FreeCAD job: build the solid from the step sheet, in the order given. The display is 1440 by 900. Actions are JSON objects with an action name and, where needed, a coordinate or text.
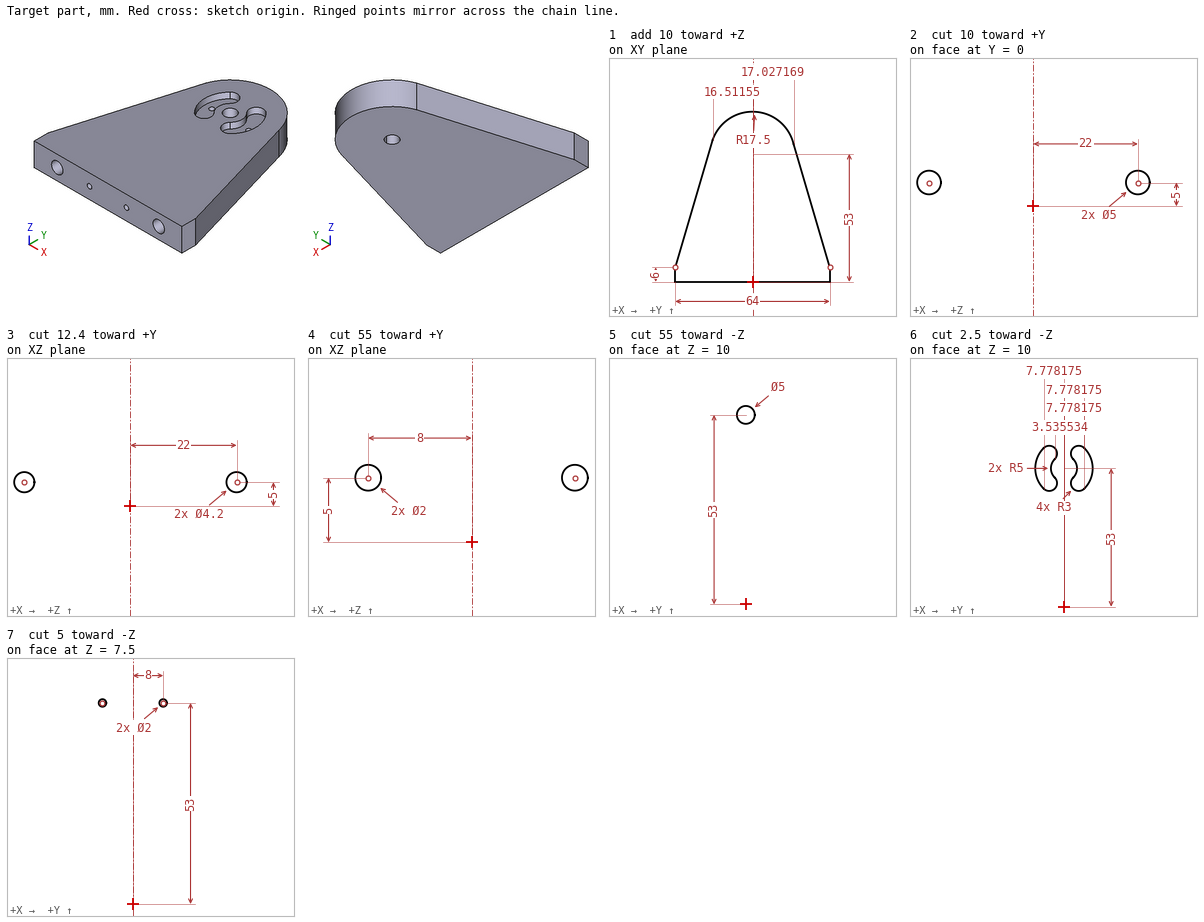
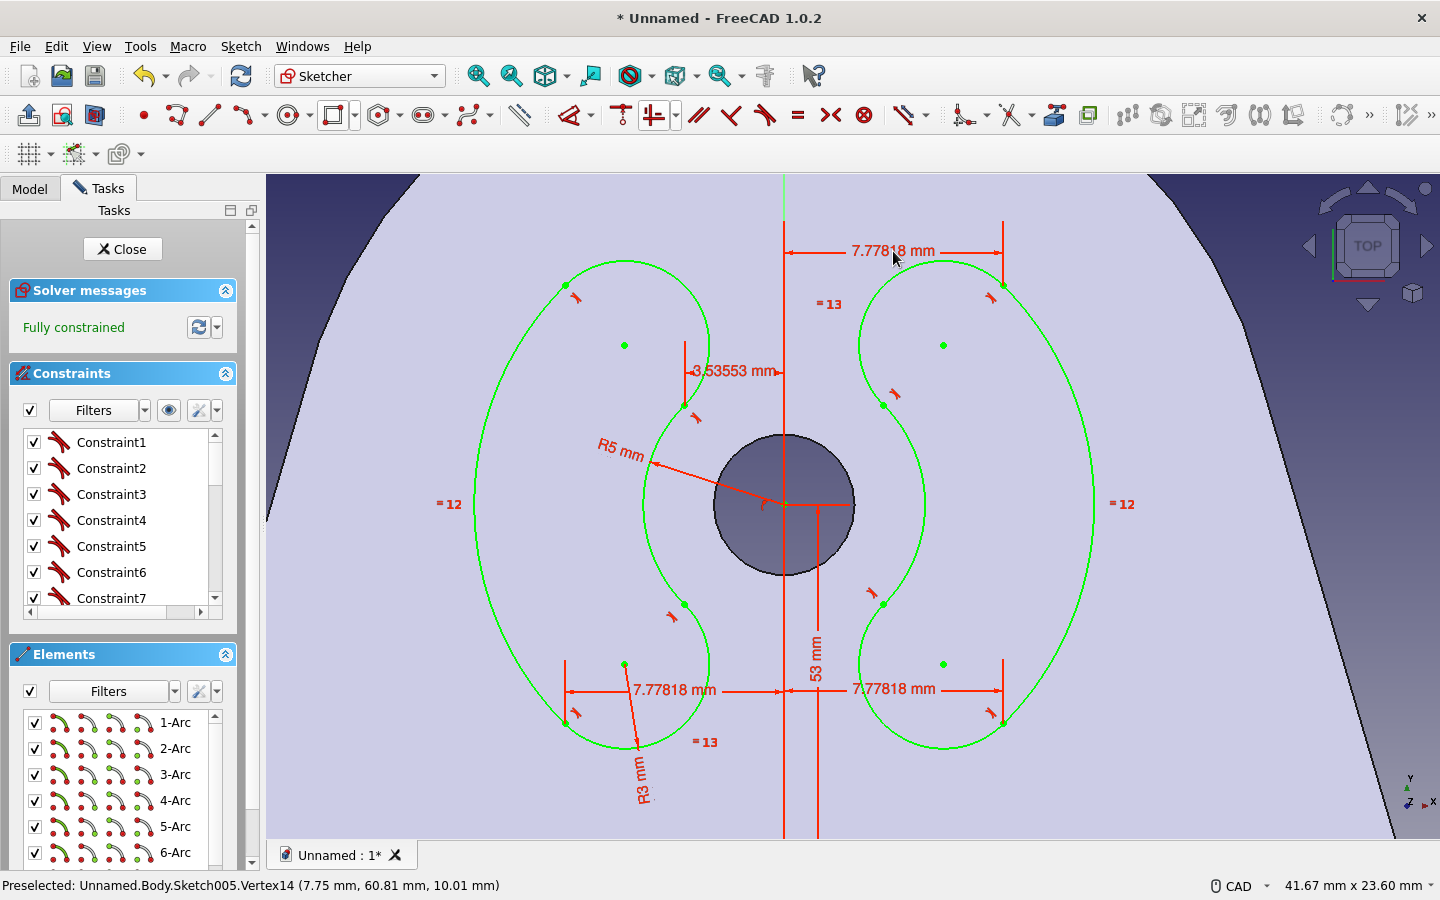
{"action": "left_click", "coordinate": [123, 249]}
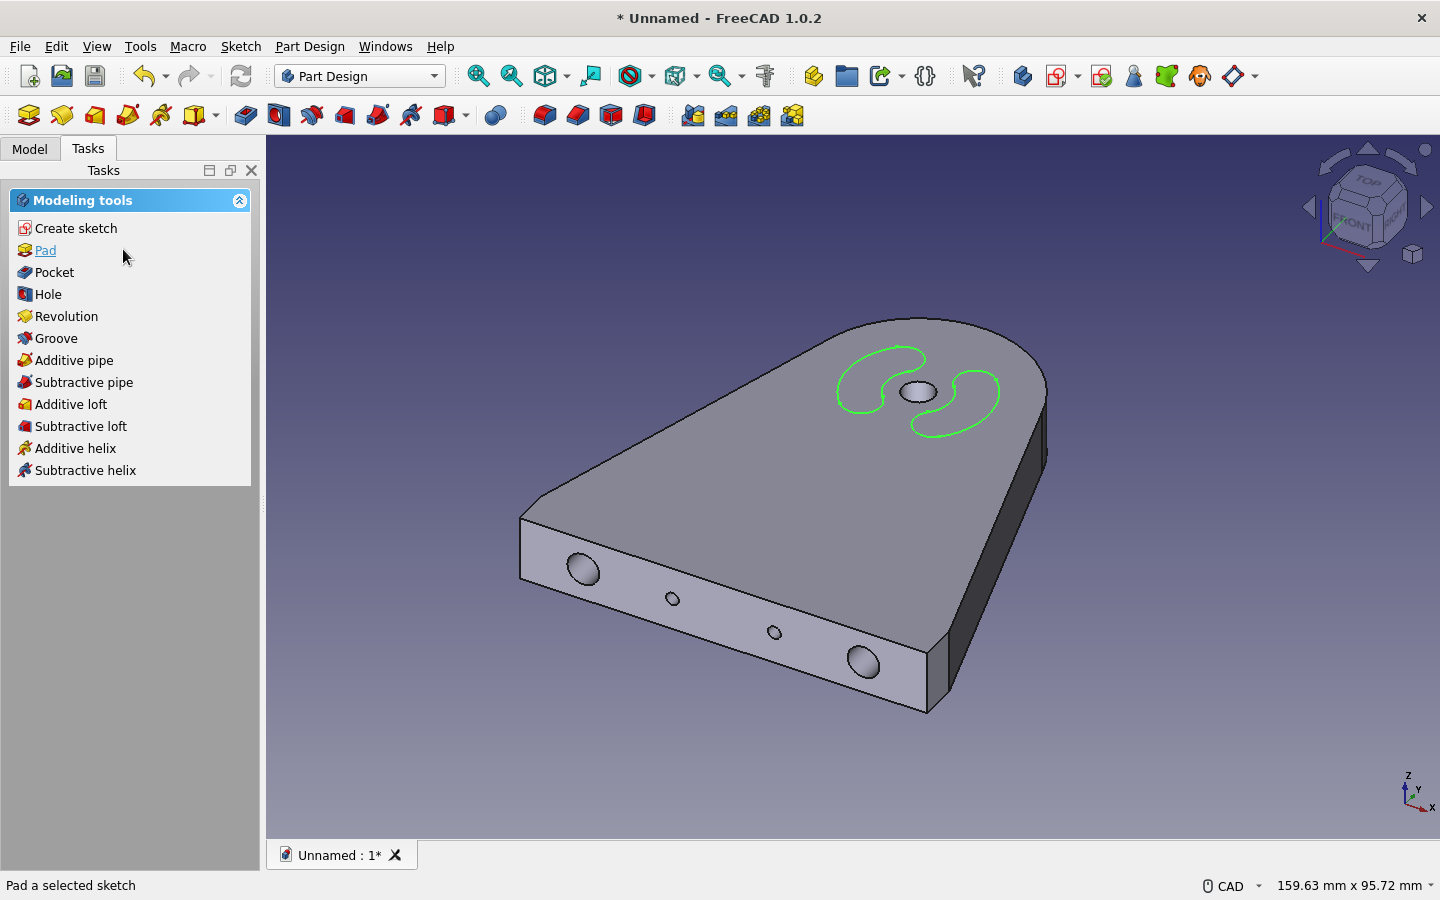
{"action": "left_click", "coordinate": [246, 116]}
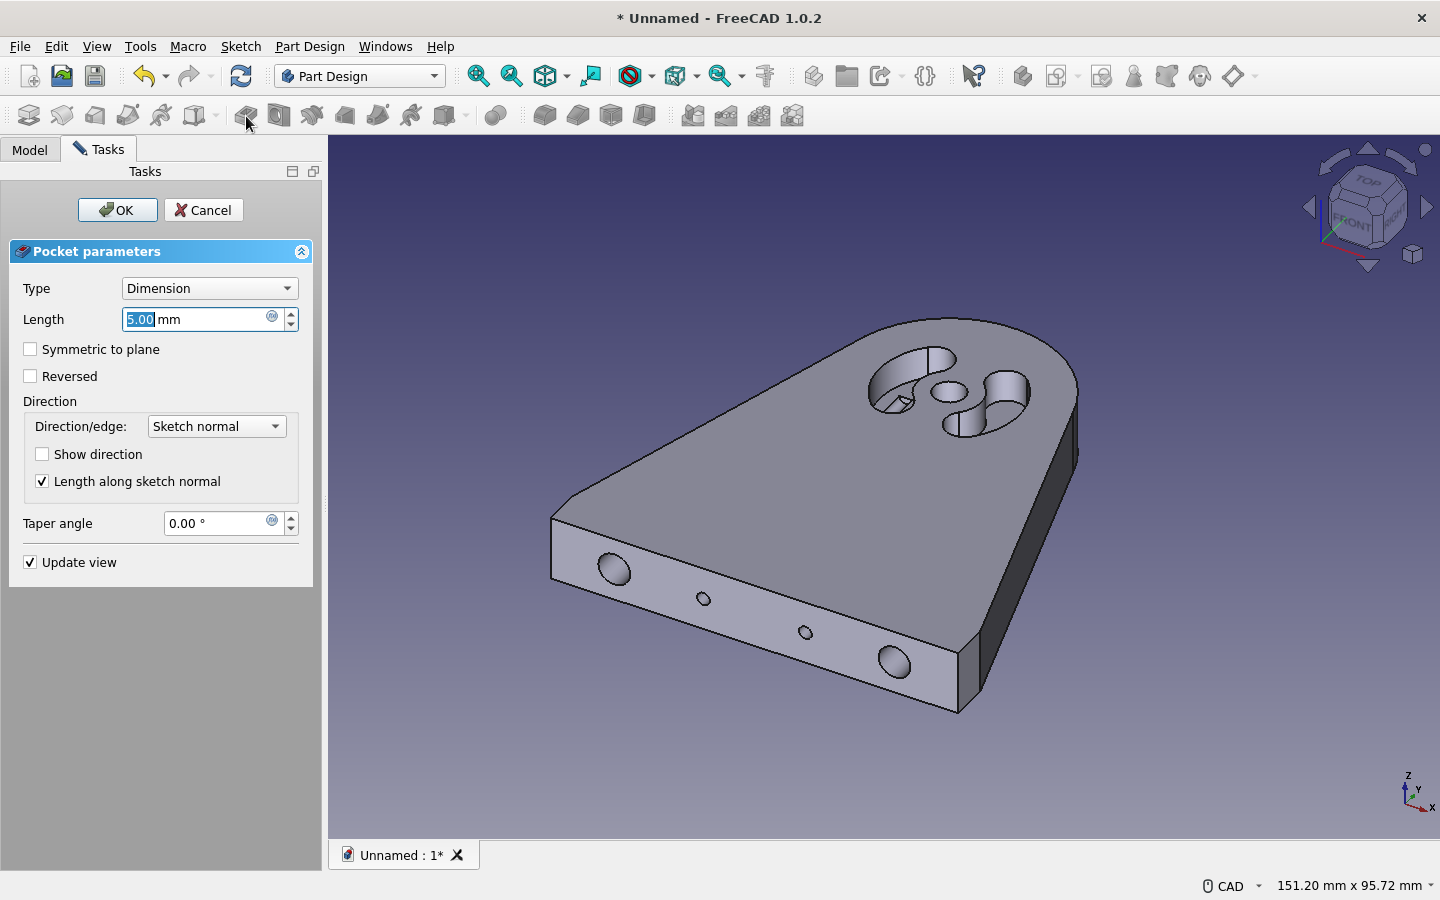
{"action": "type", "text": "2.5"}
{"action": "key", "text": "Tab"}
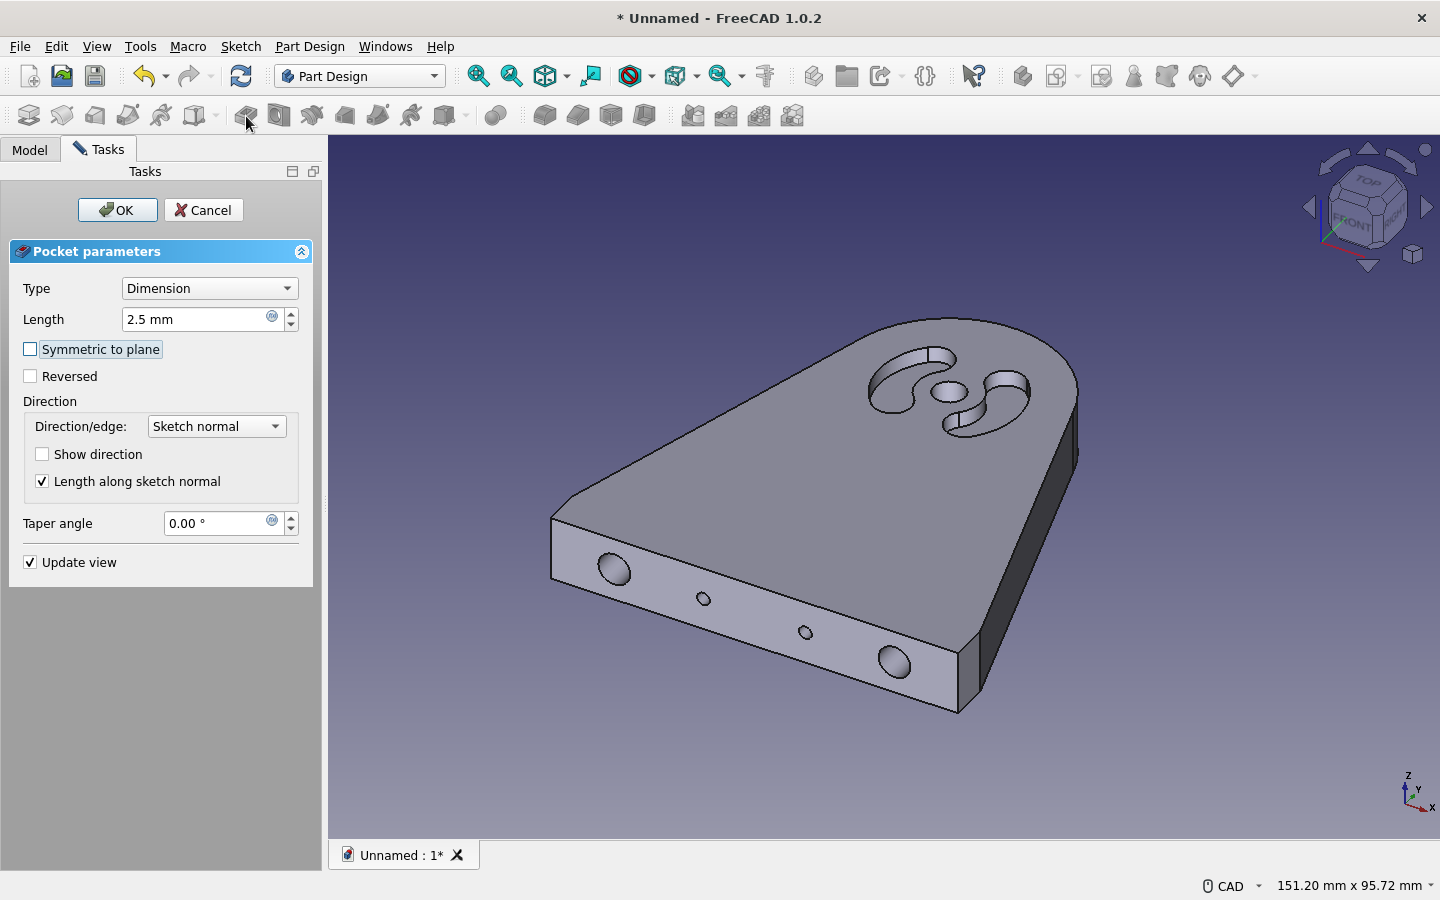
{"action": "left_click", "coordinate": [118, 210]}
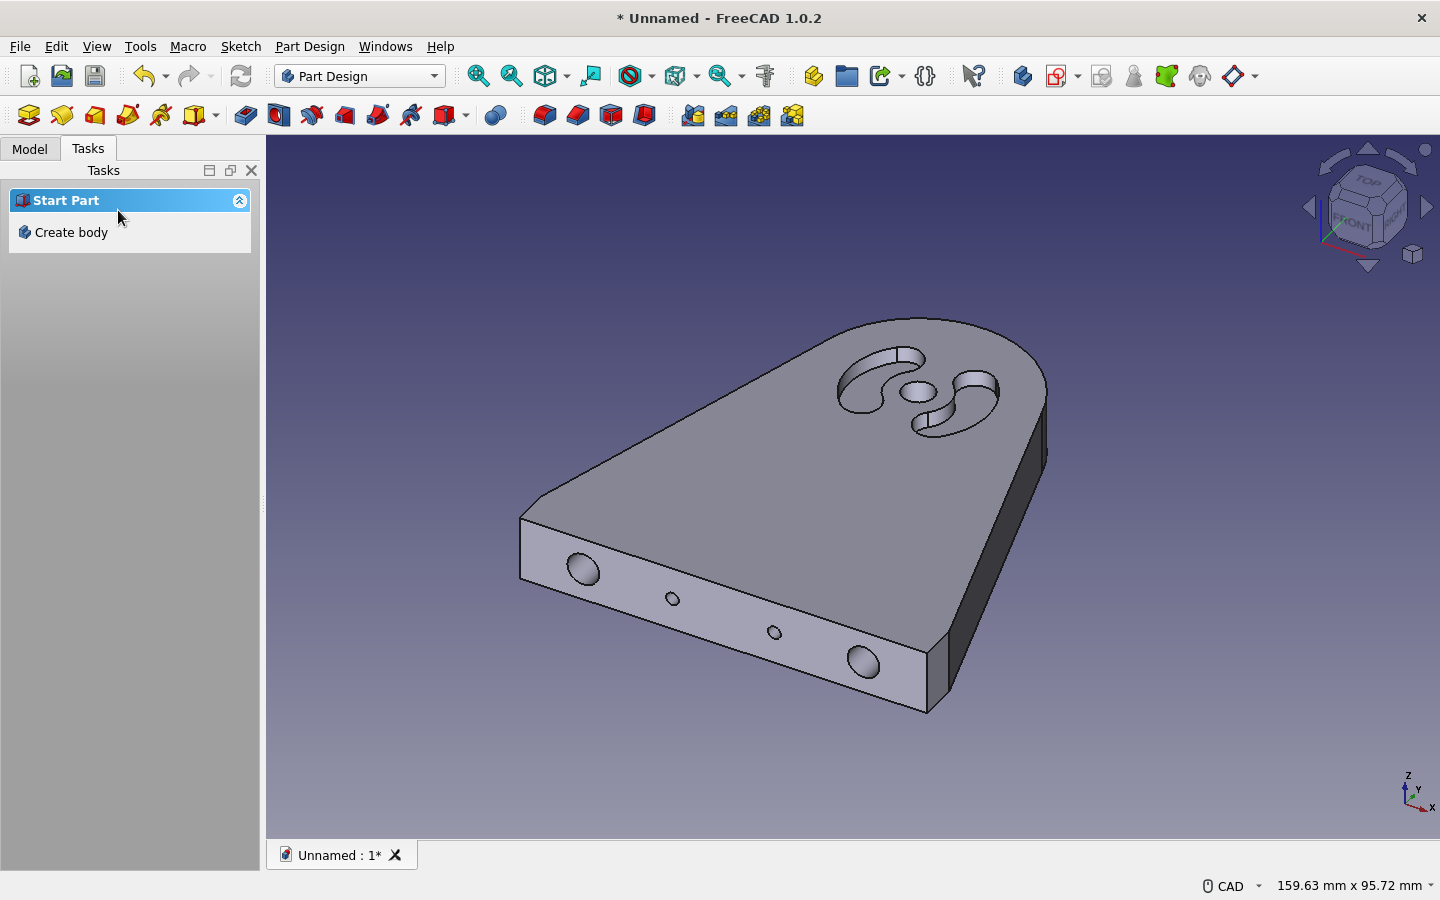
{"action": "left_click", "coordinate": [867, 389]}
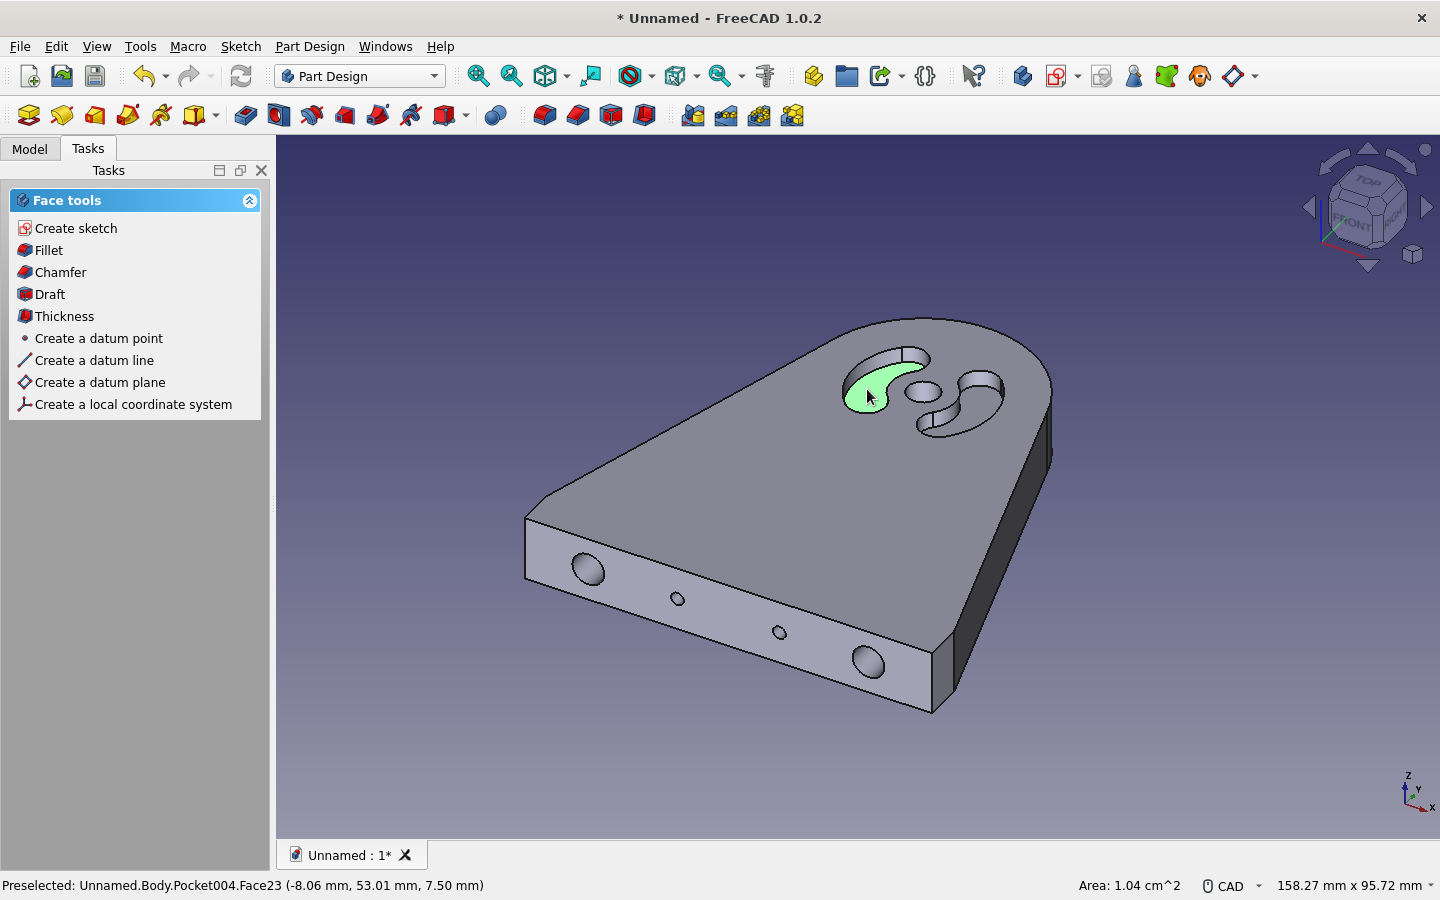
{"action": "left_click", "coordinate": [1056, 76]}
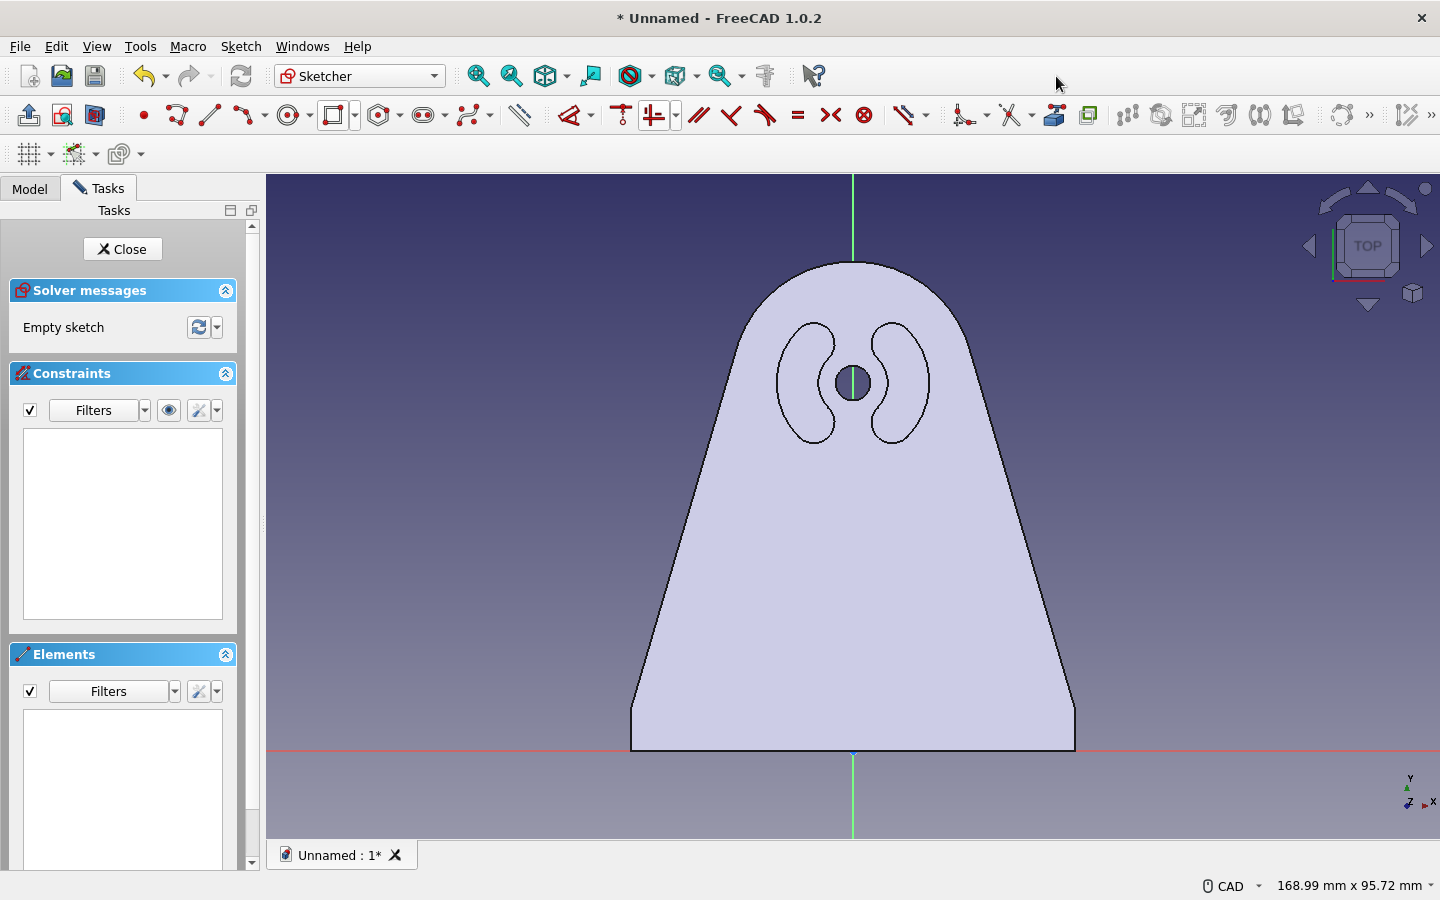
{"action": "scroll", "coordinate": [867, 359], "scroll_direction": "up", "scroll_amount": 9}